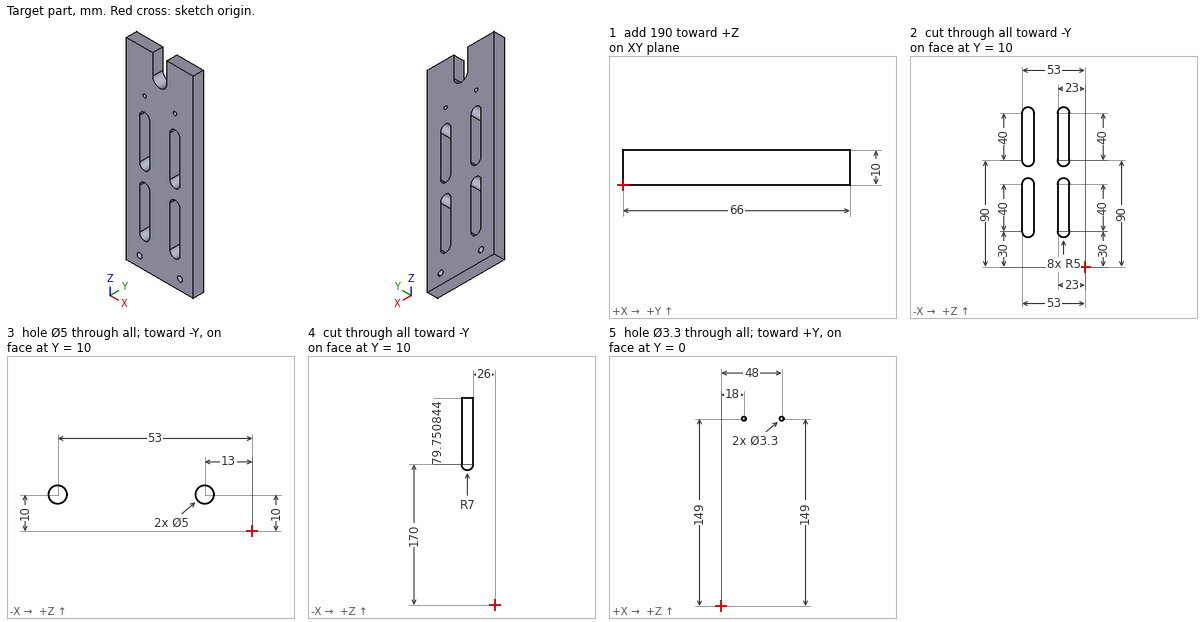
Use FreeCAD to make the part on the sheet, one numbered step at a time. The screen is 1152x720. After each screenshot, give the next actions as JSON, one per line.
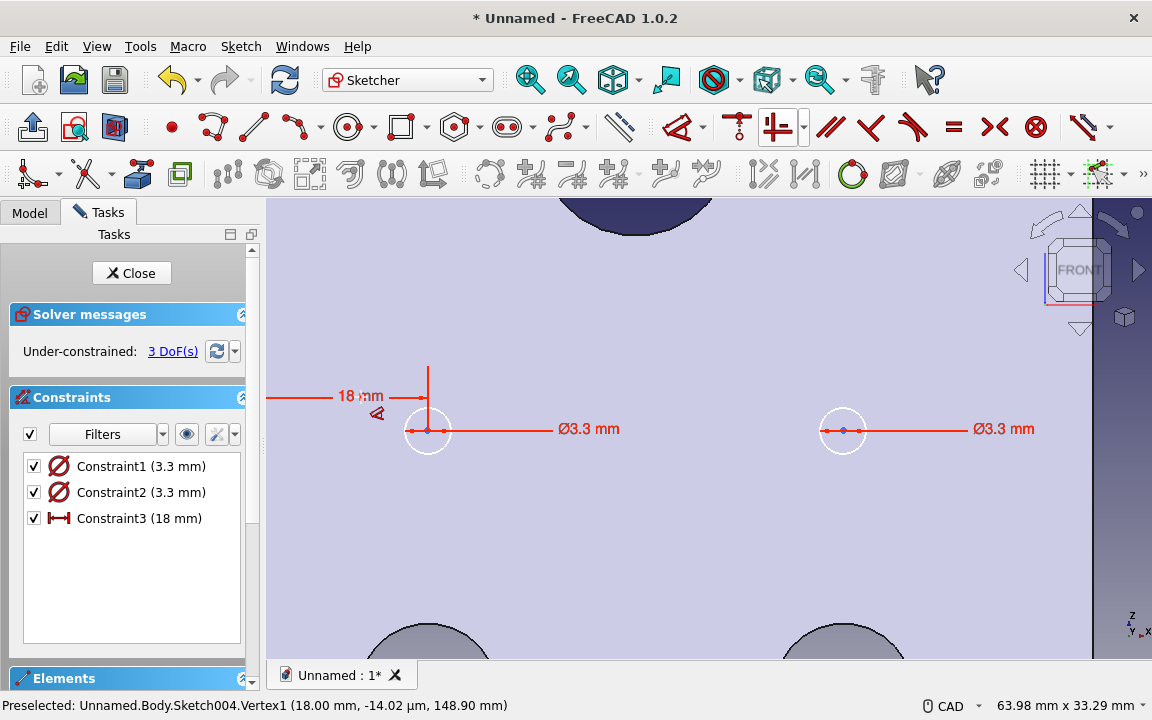
{"action": "left_click", "coordinate": [843, 431]}
{"action": "left_click", "coordinate": [568, 397]}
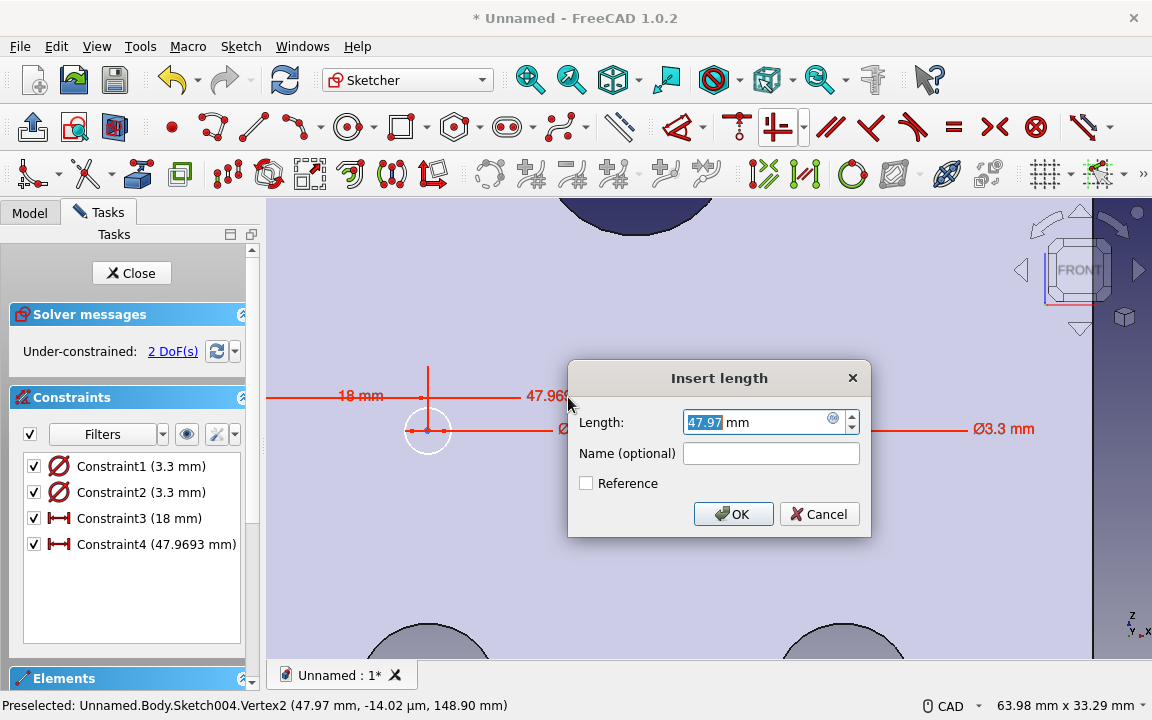
{"action": "type", "text": "48"}
{"action": "key", "text": "Return"}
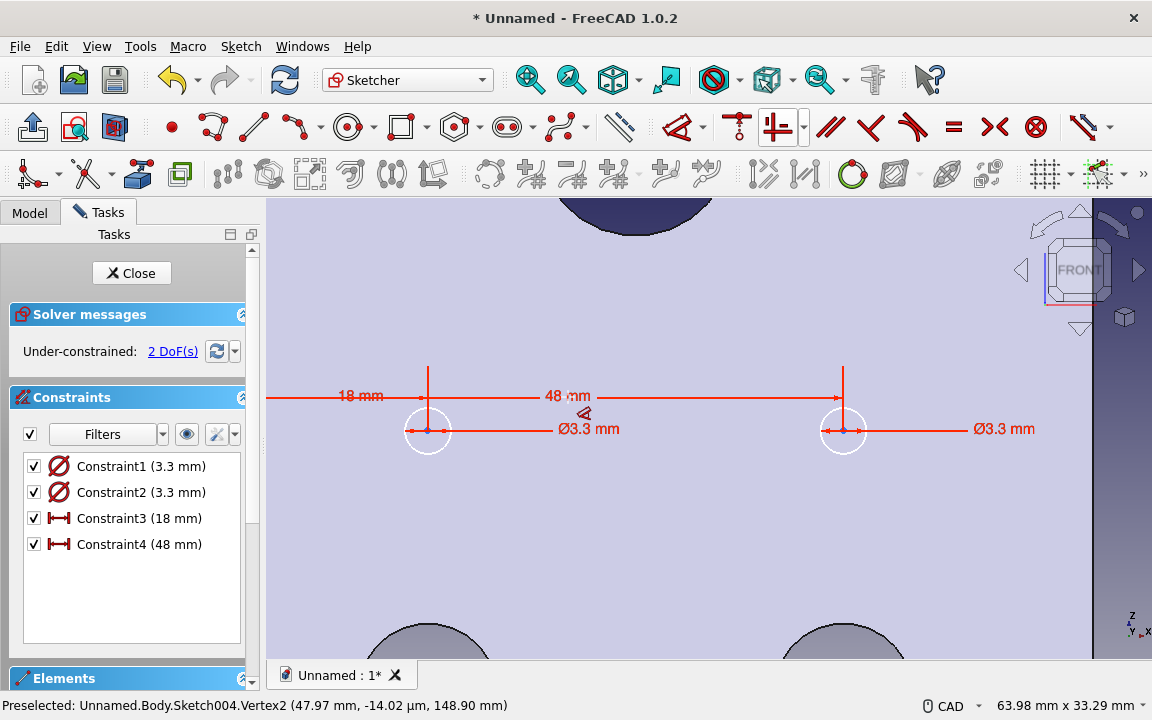
{"action": "left_click", "coordinate": [428, 431]}
{"action": "left_click", "coordinate": [462, 531]}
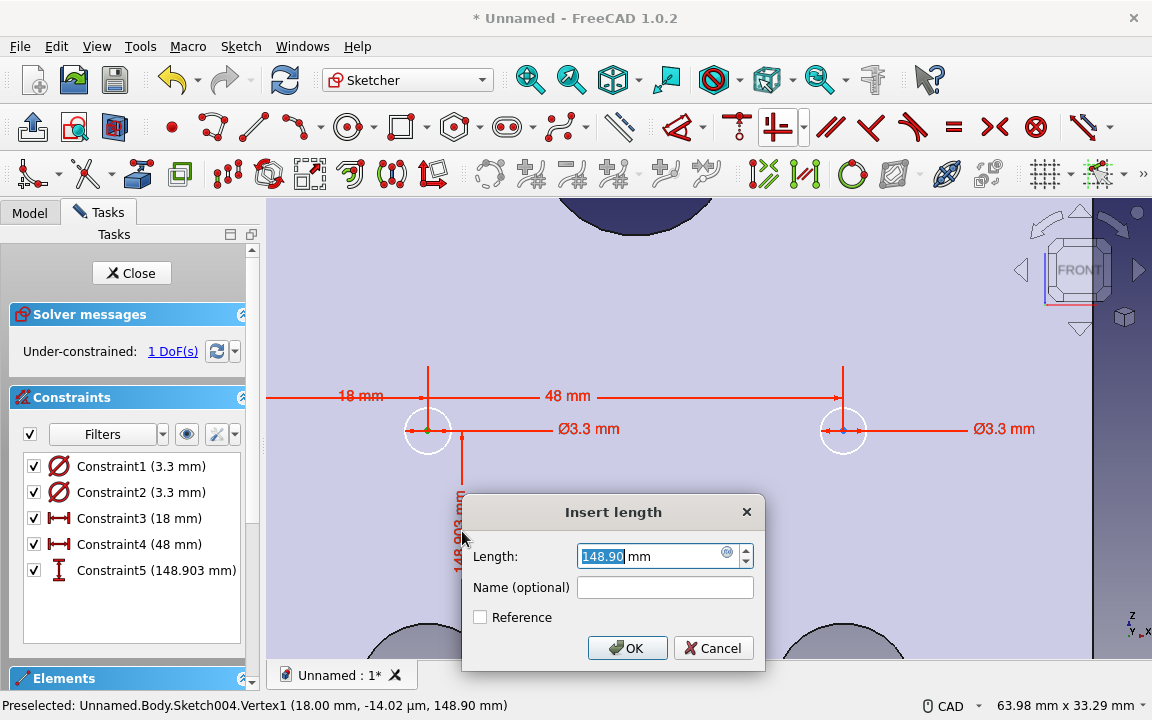
{"action": "type", "text": "149"}
{"action": "key", "text": "Return"}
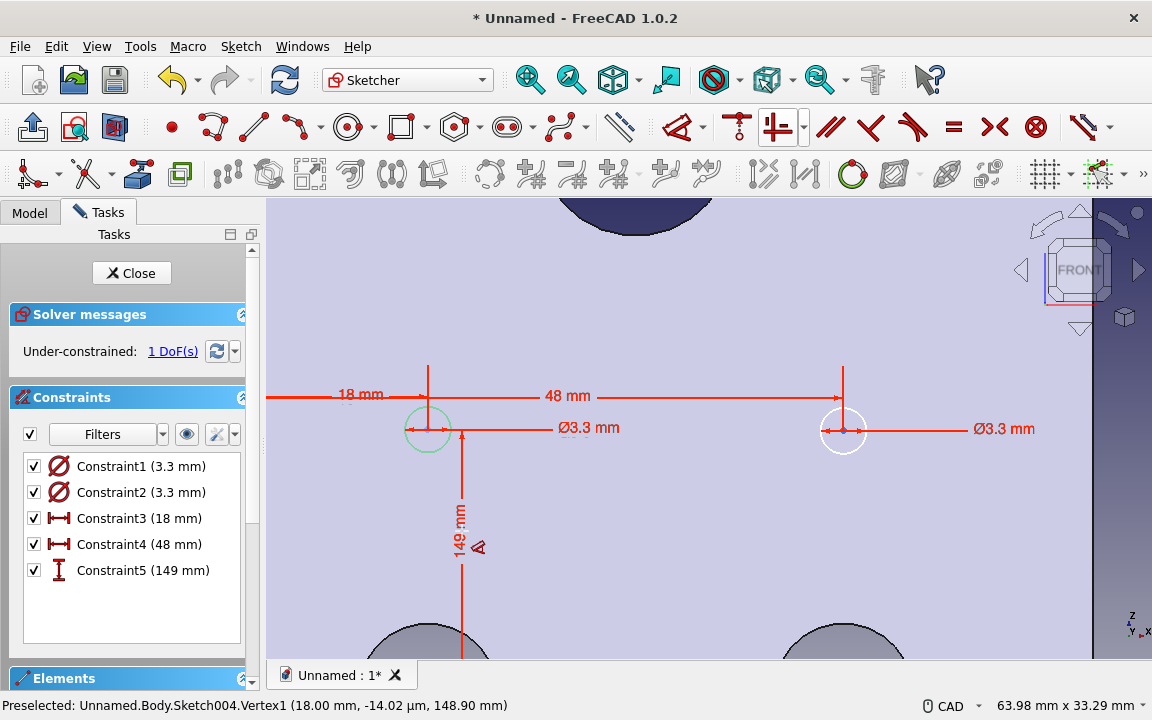
{"action": "left_click", "coordinate": [843, 431]}
{"action": "left_click", "coordinate": [877, 531]}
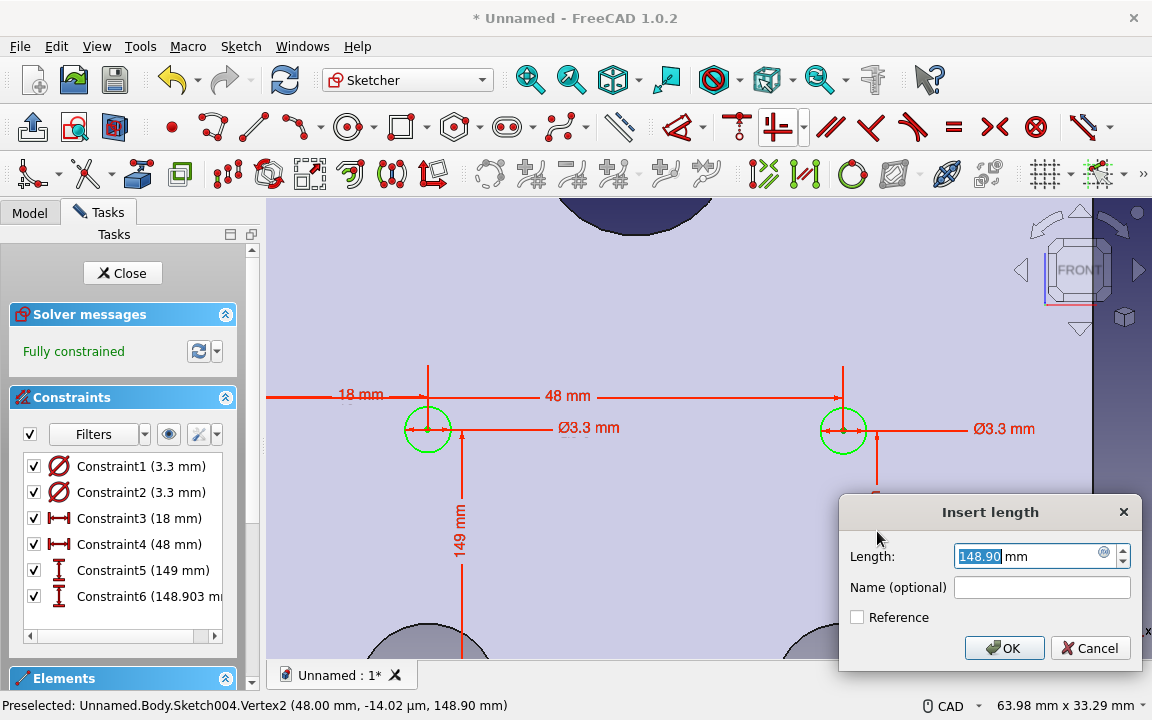
{"action": "type", "text": "149"}
{"action": "key", "text": "Return"}
{"action": "key", "text": "Escape"}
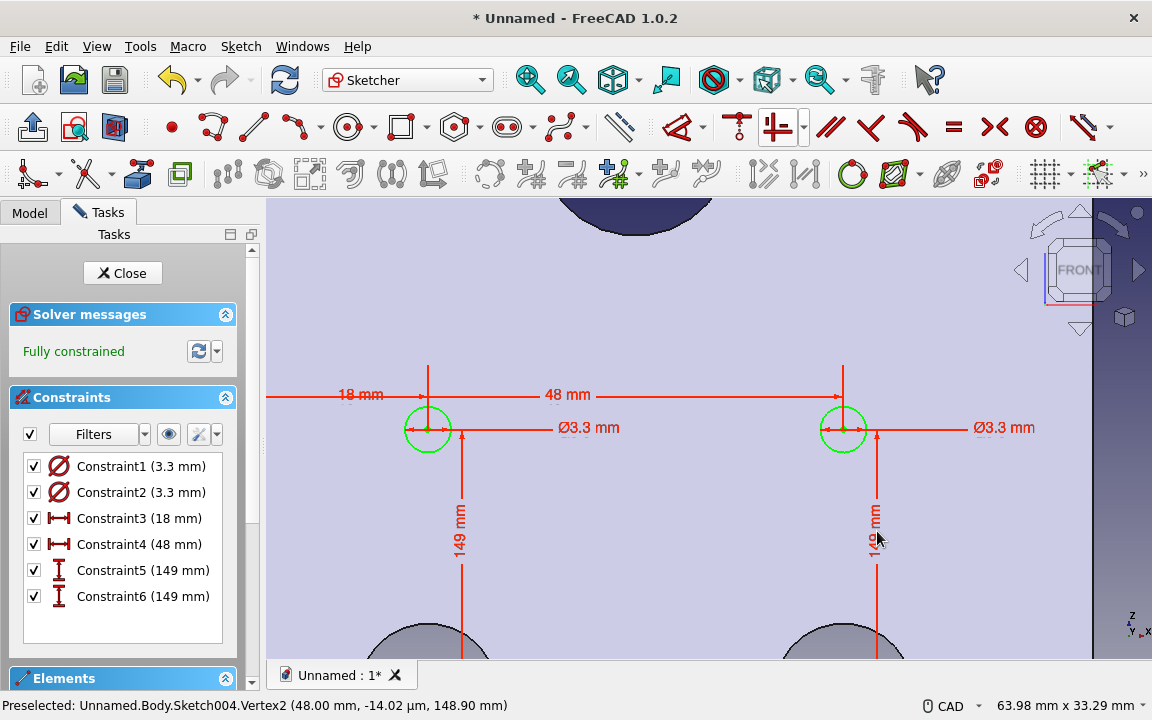
{"action": "left_click", "coordinate": [123, 273]}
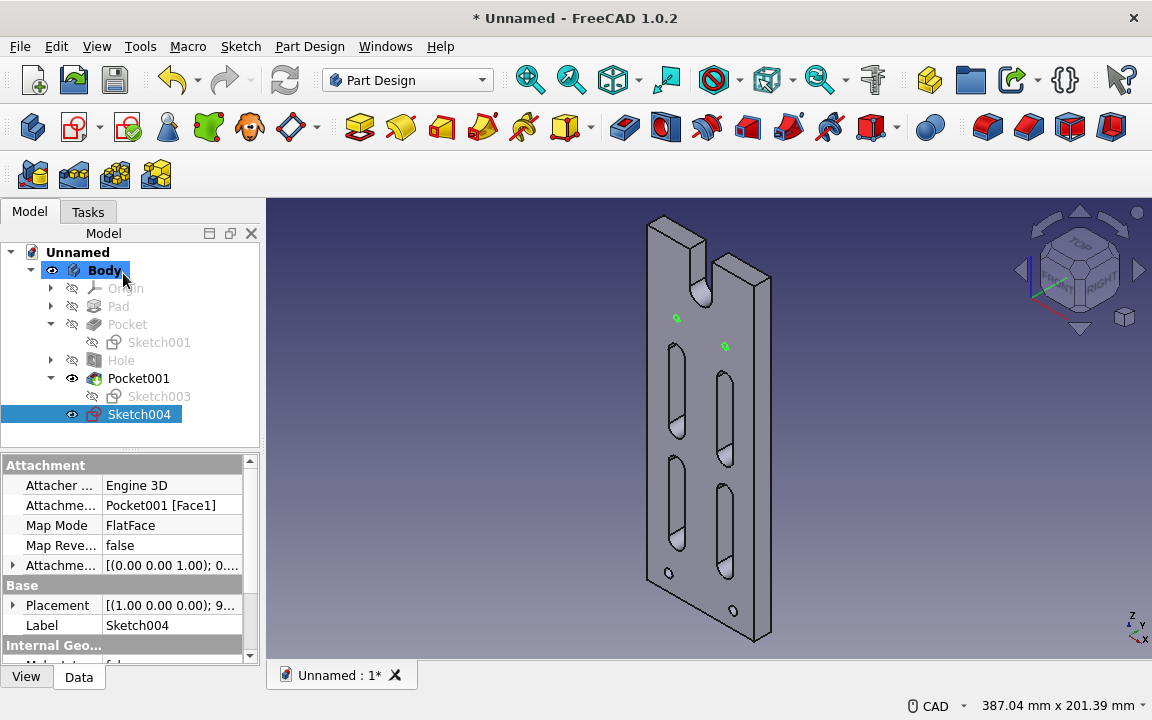
{"action": "left_click", "coordinate": [666, 128]}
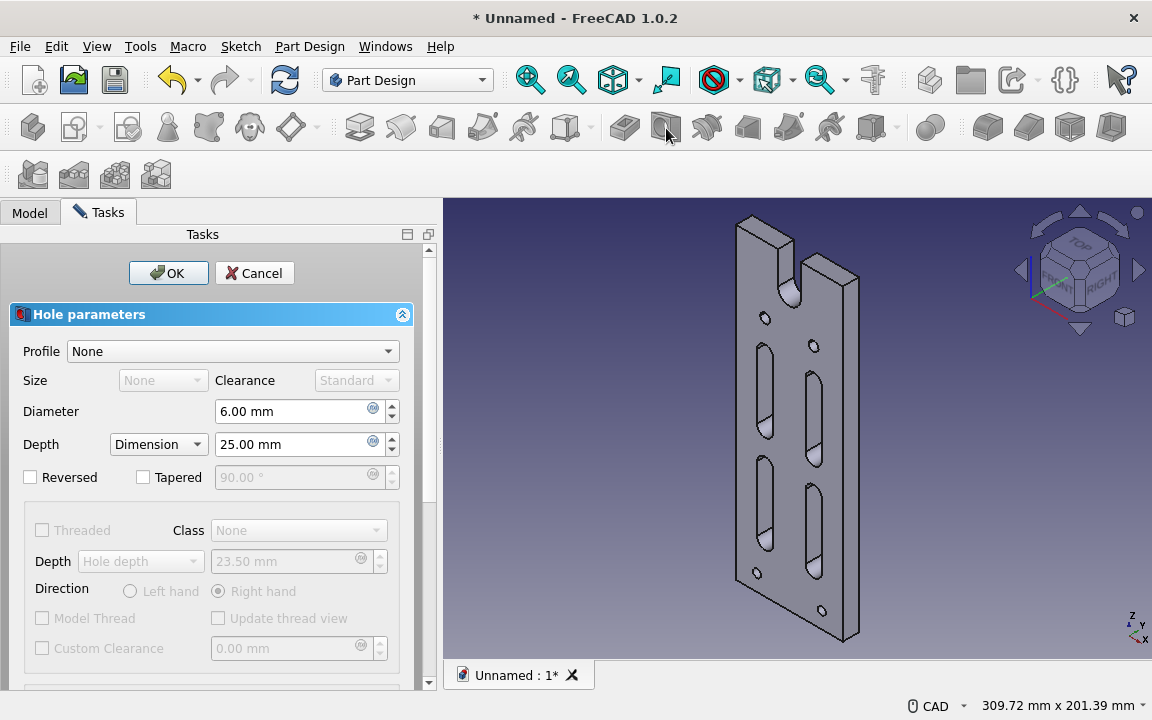
{"action": "triple_click", "coordinate": [300, 412]}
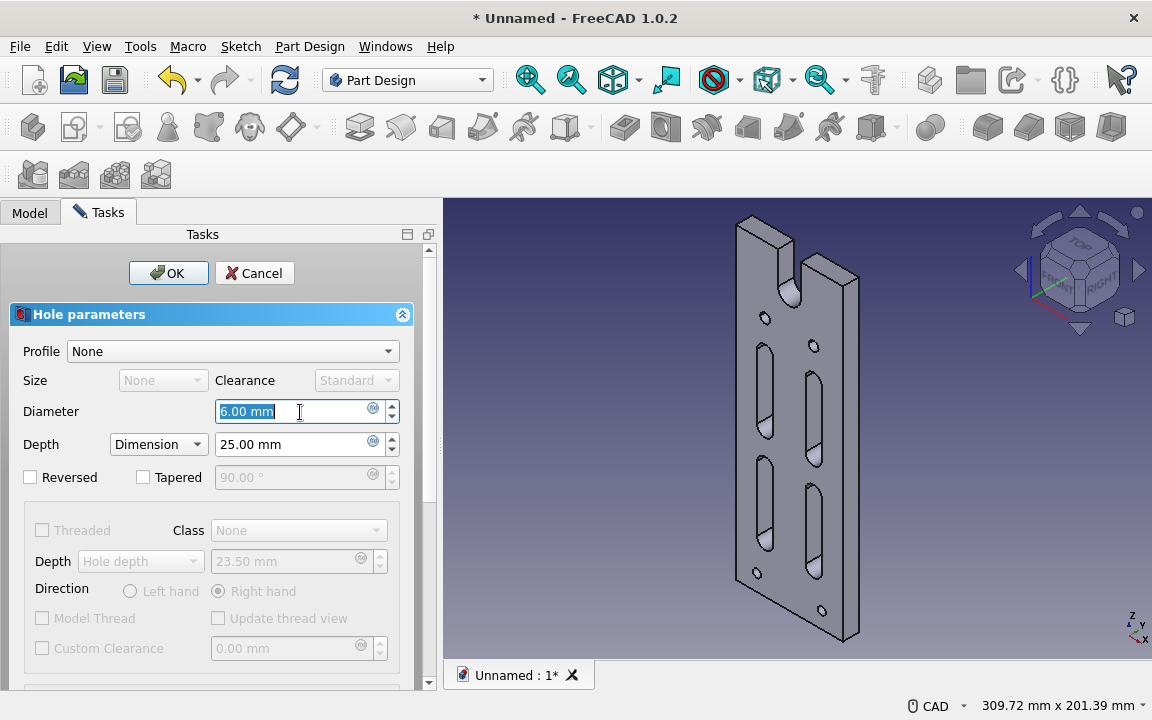
{"action": "type", "text": "3.3"}
{"action": "key", "text": "Tab"}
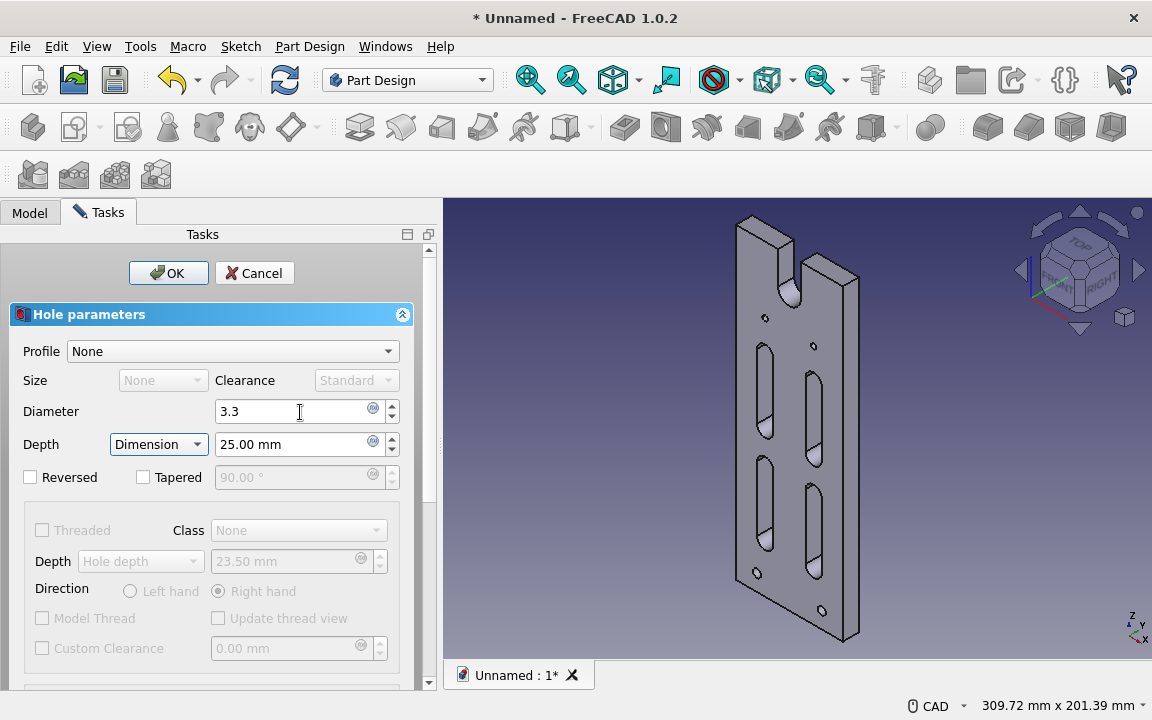
{"action": "left_click", "coordinate": [160, 444]}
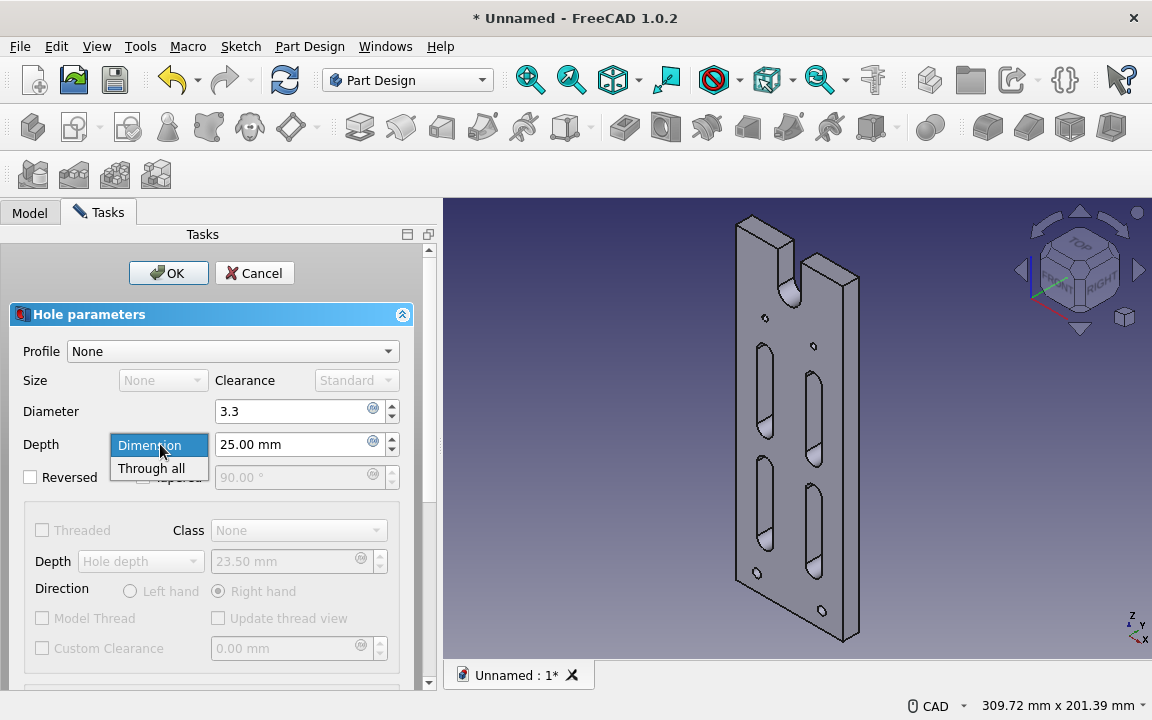
{"action": "left_click", "coordinate": [158, 468]}